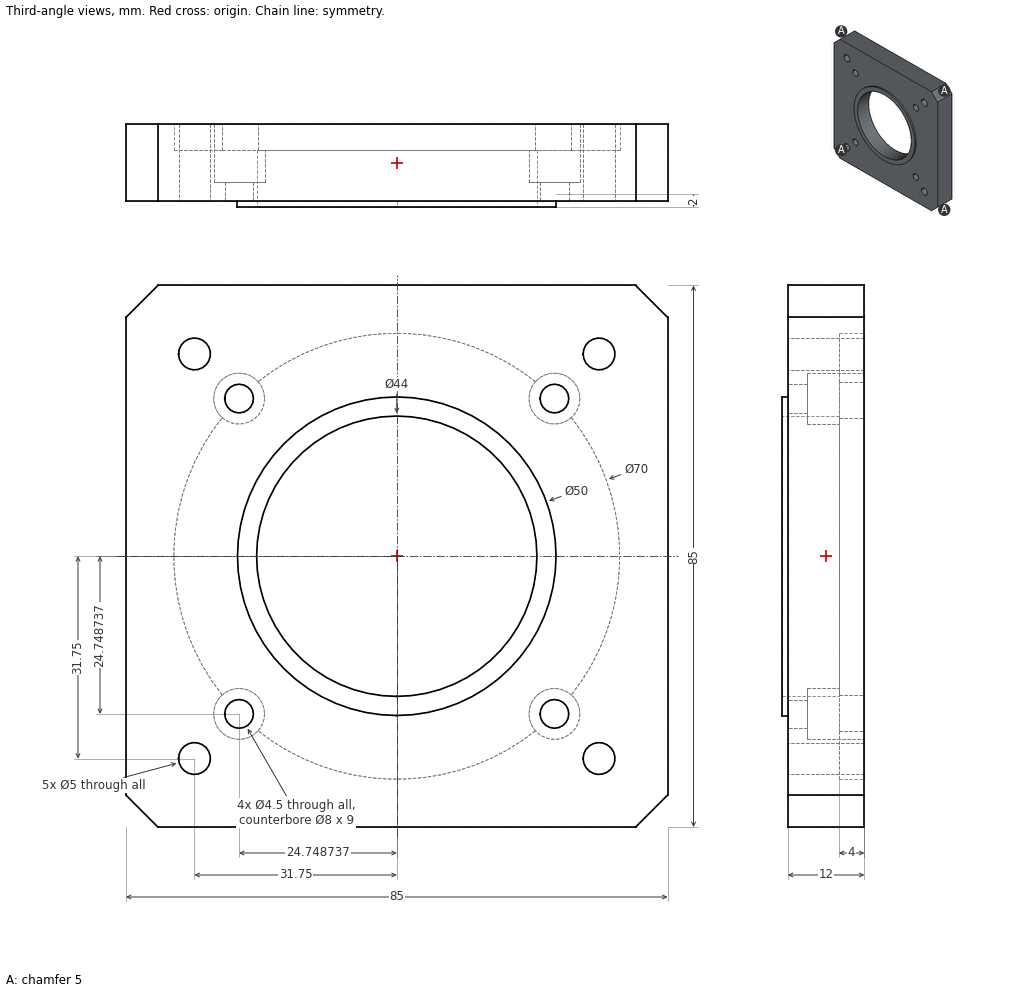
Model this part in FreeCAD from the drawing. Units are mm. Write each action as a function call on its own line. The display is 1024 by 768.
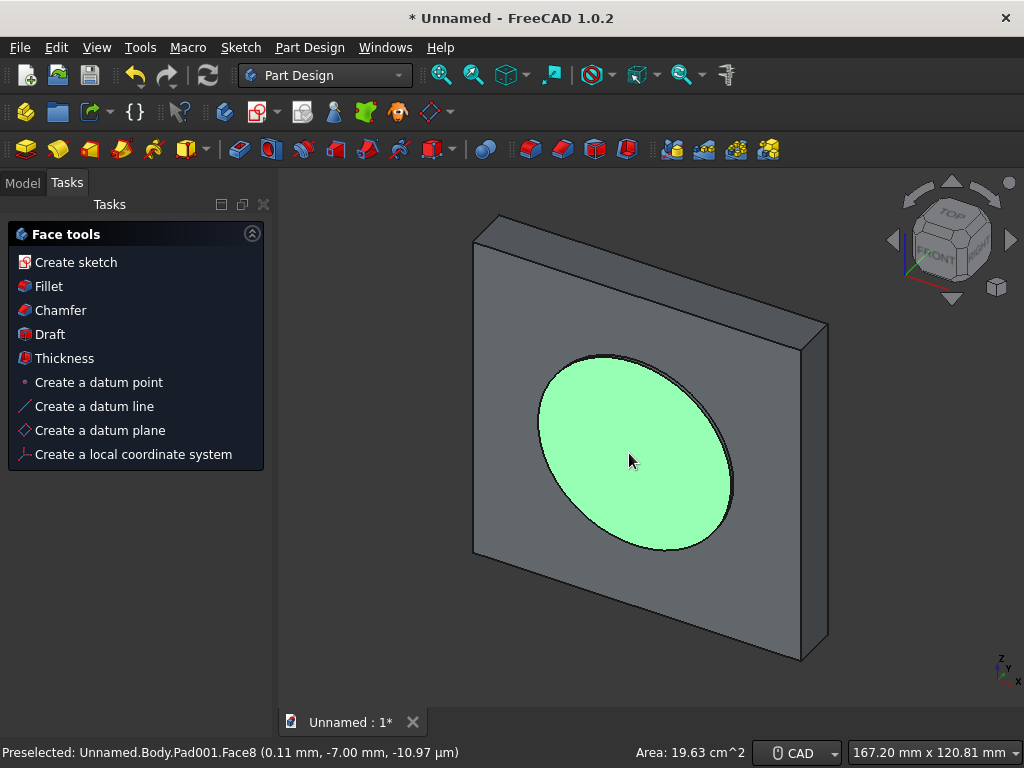
click(258, 112)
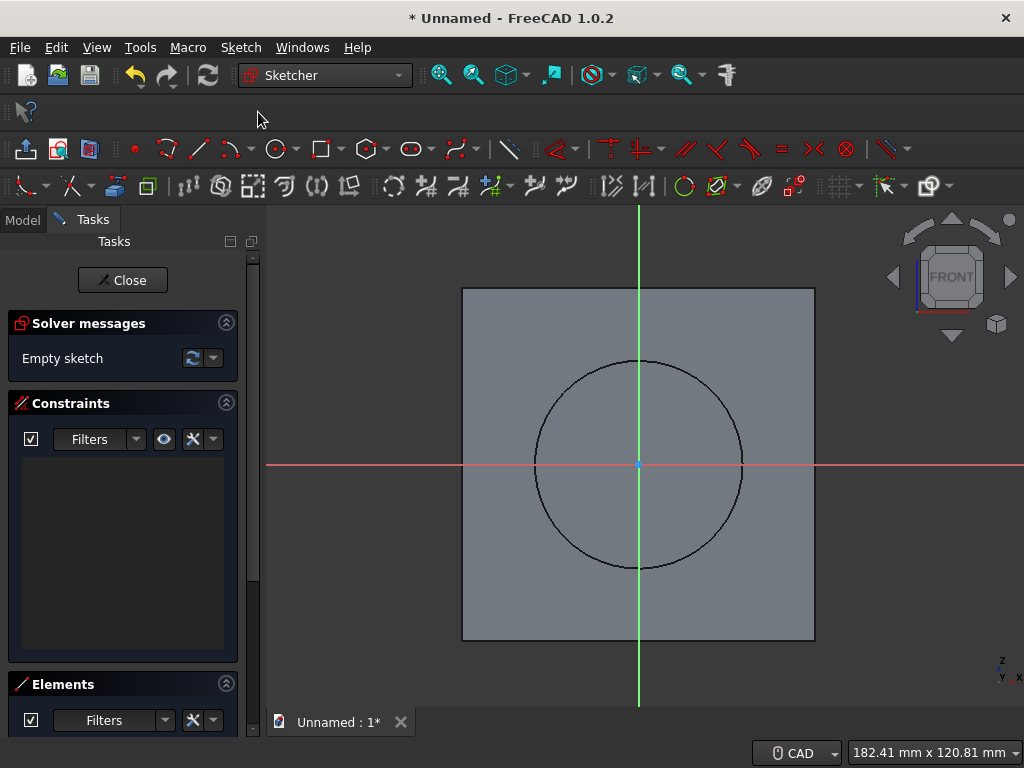
scroll(714, 475, up, 3)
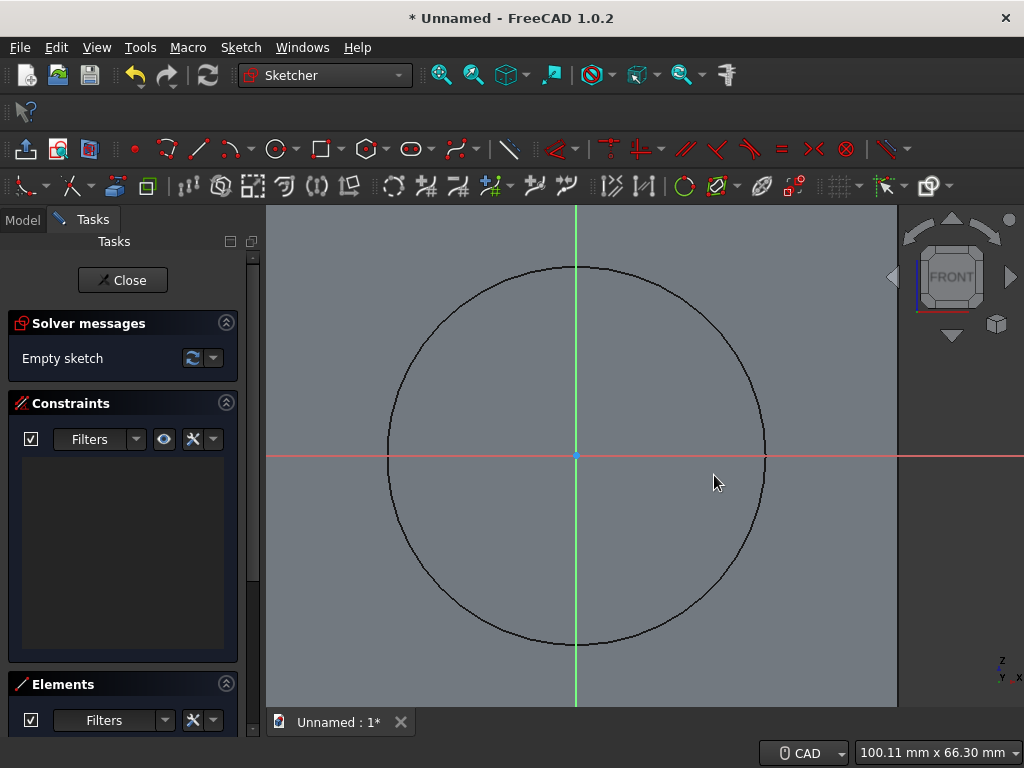
key(g)
key(c)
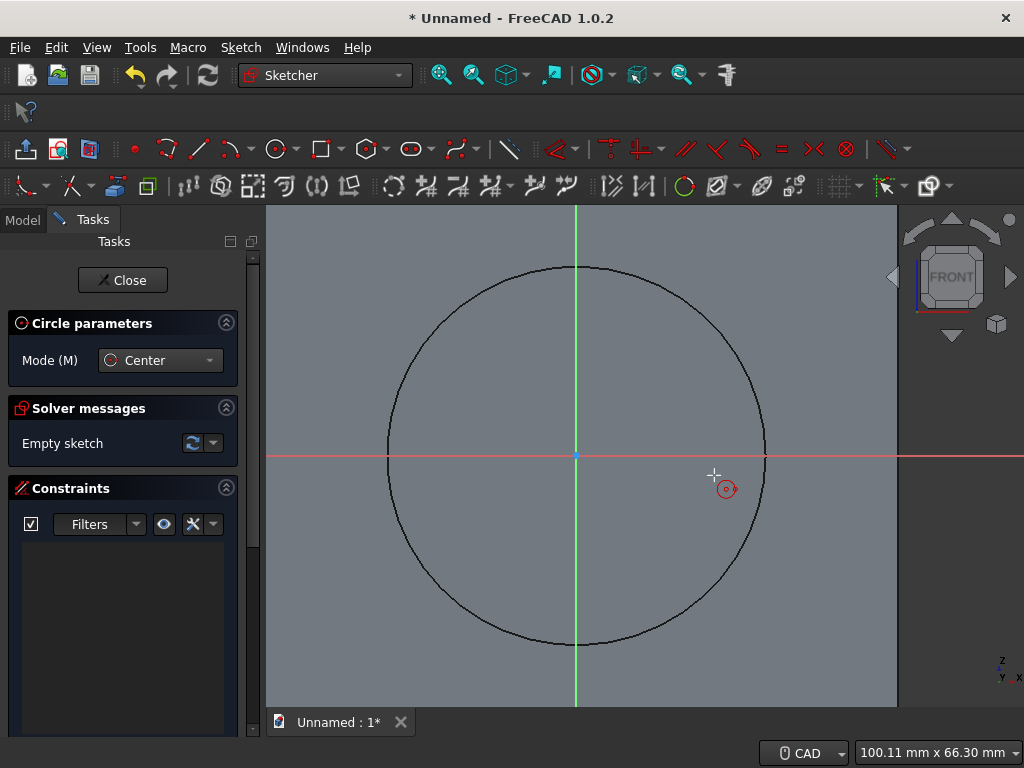
click(576, 456)
move(694, 338)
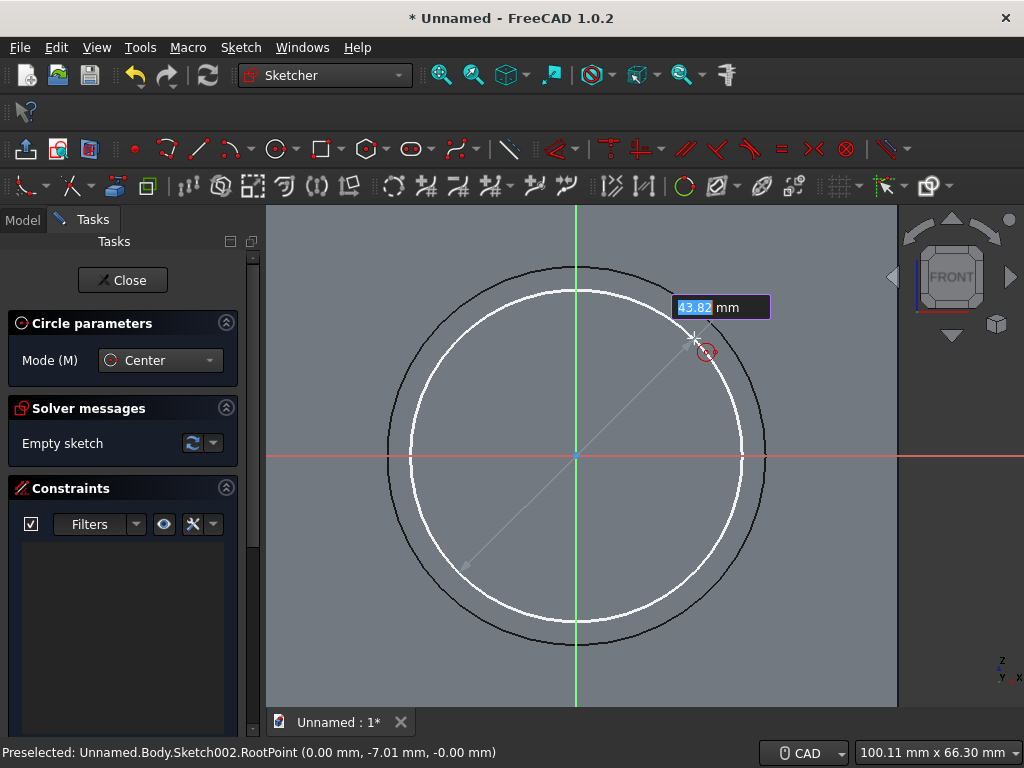
text(44)
key(Return)
key(Escape)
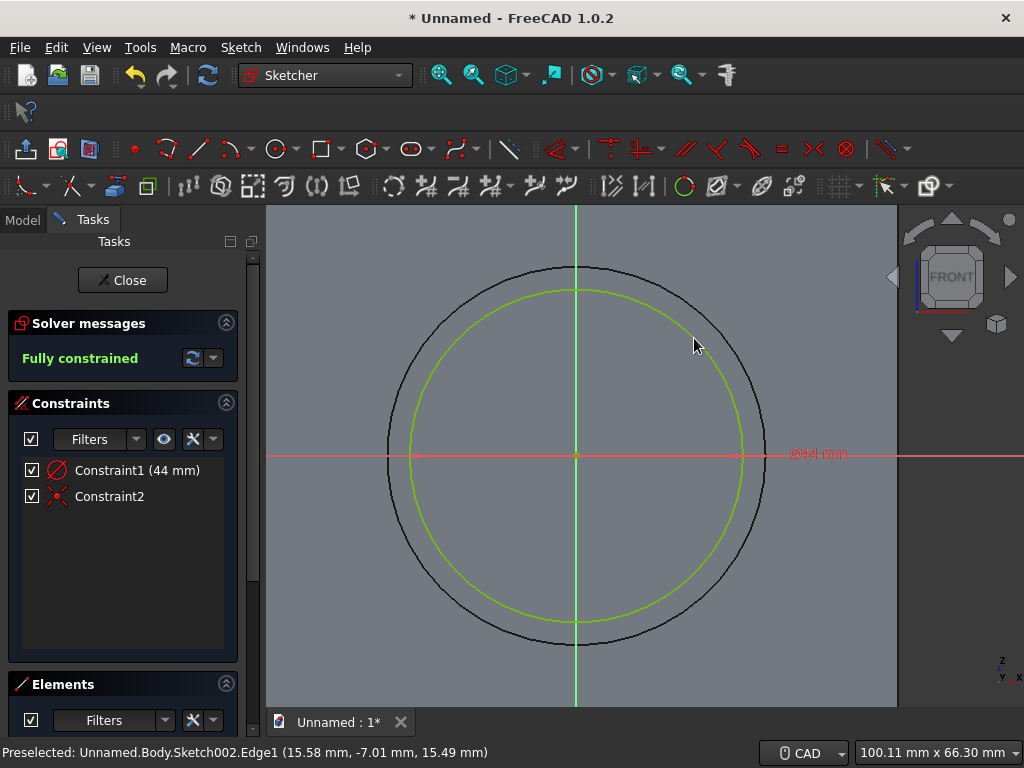
click(123, 280)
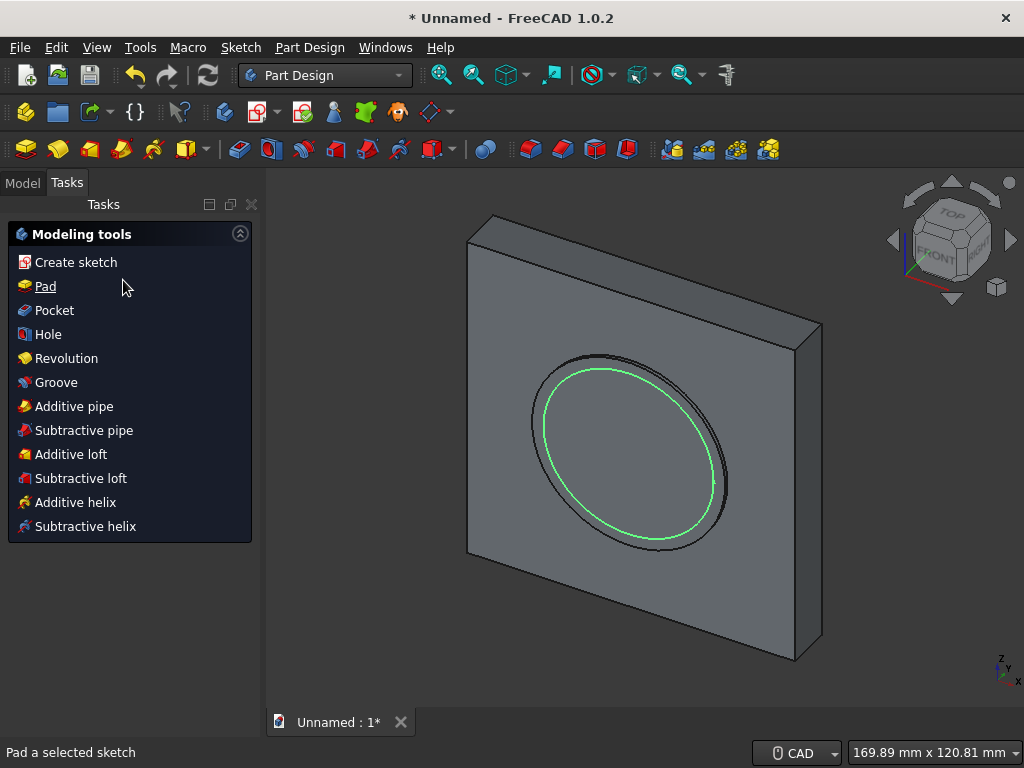
click(240, 150)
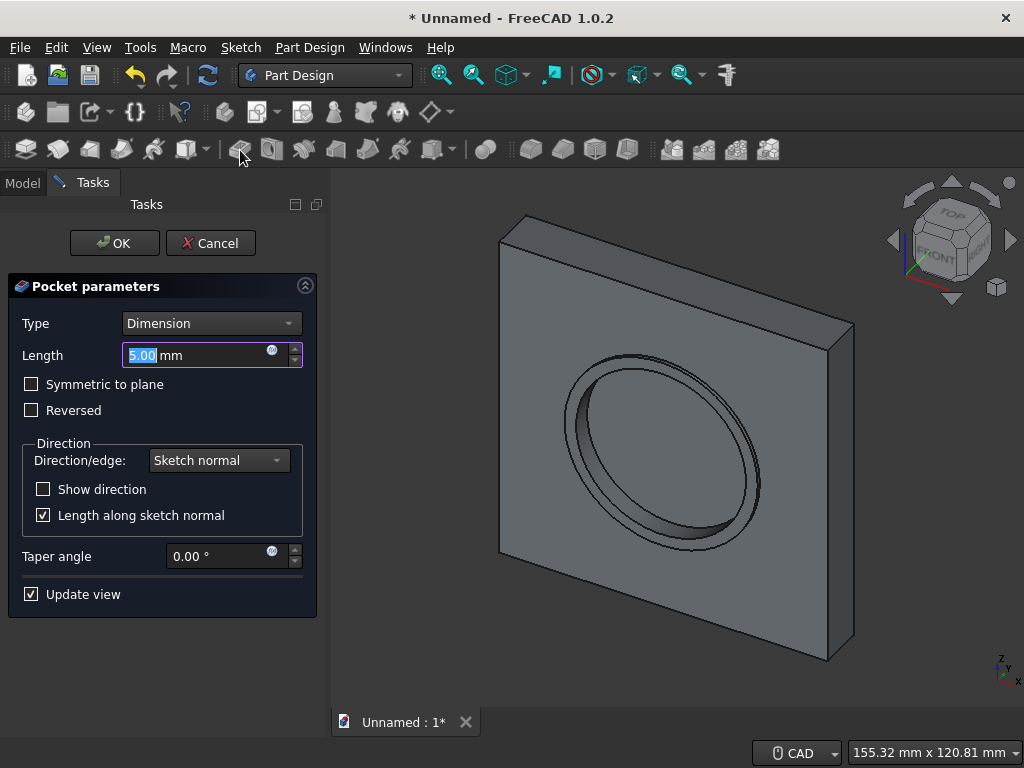
click(212, 324)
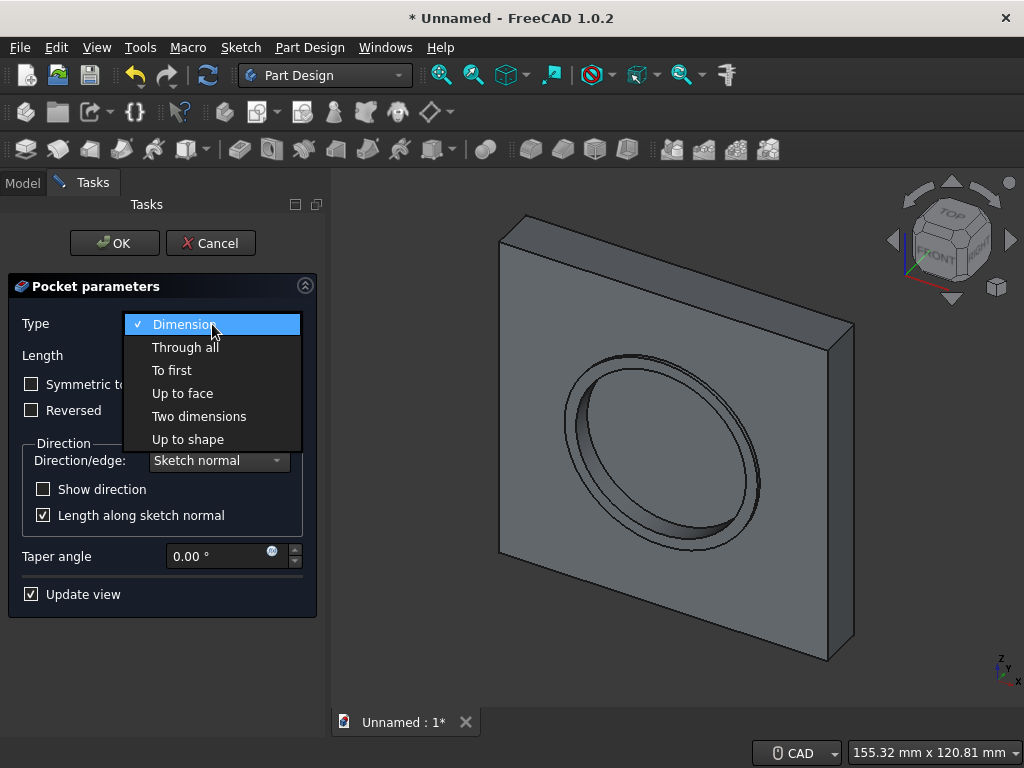
click(212, 348)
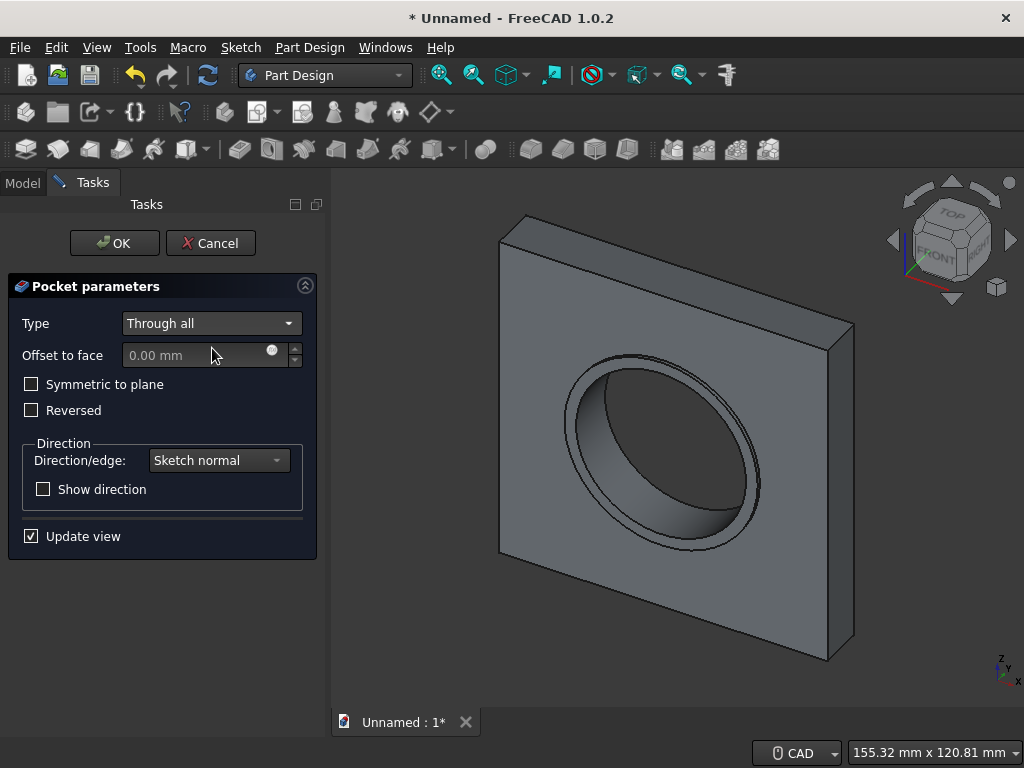
click(115, 243)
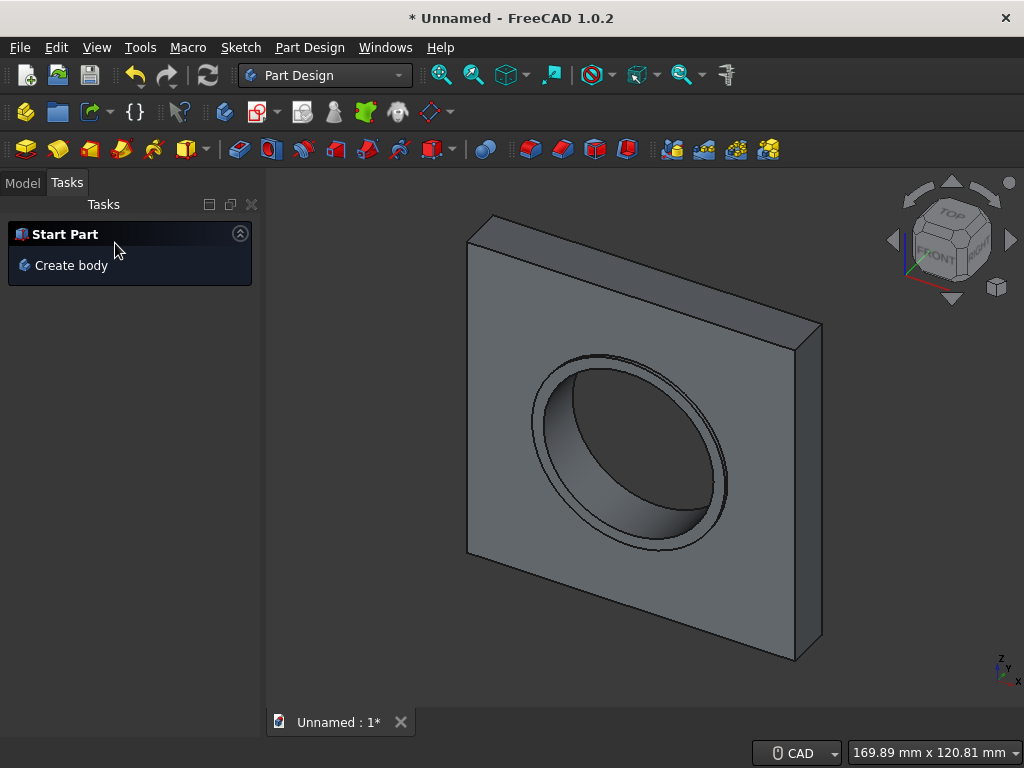
key(4)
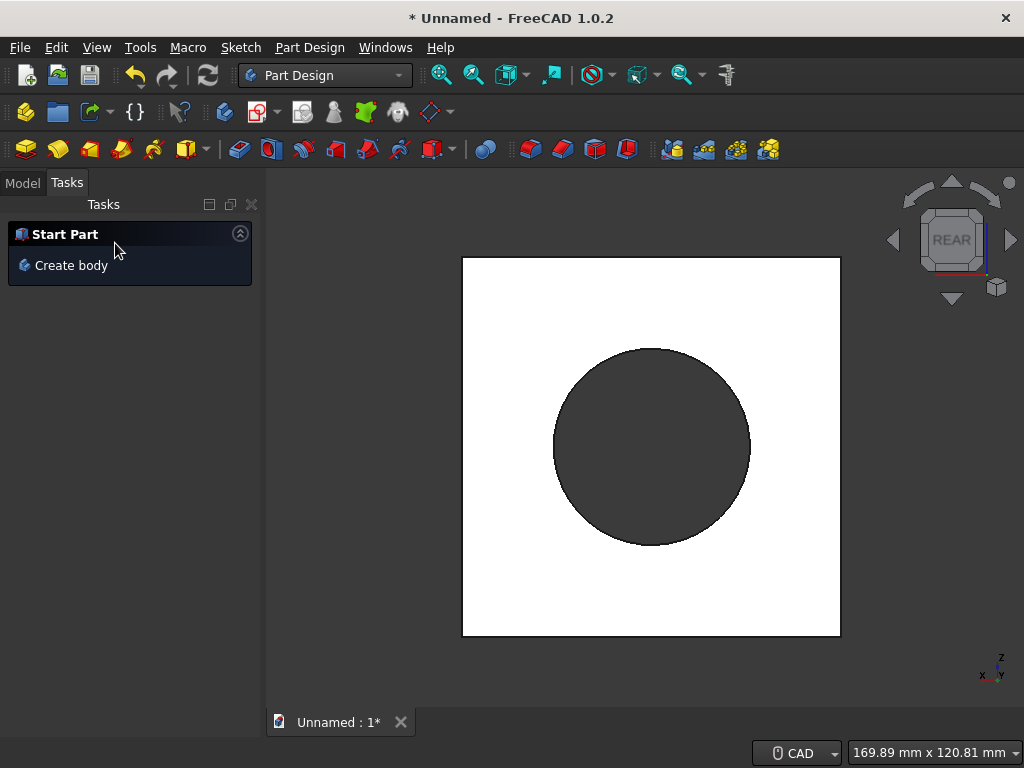
click(543, 338)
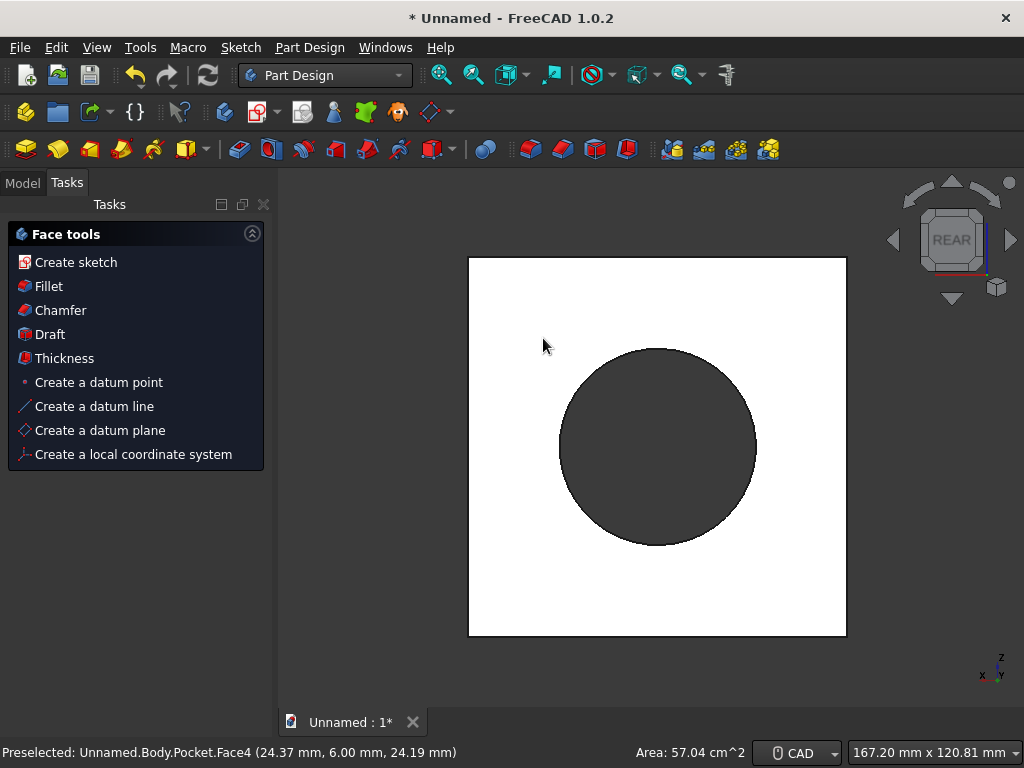
click(258, 112)